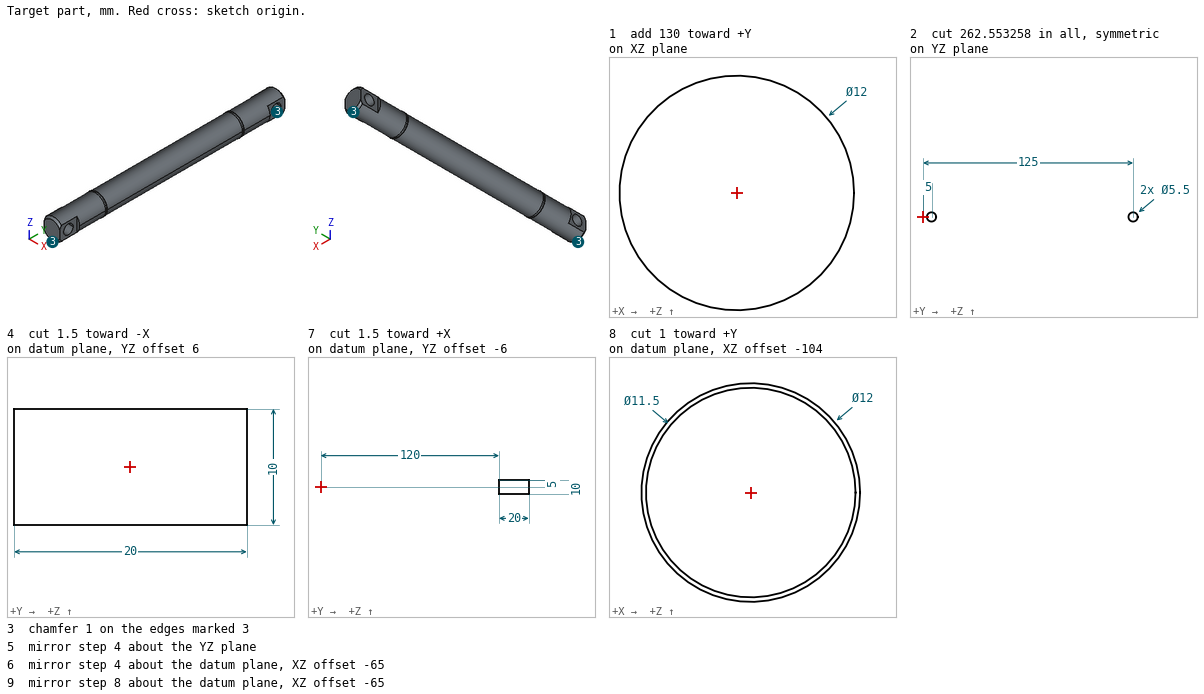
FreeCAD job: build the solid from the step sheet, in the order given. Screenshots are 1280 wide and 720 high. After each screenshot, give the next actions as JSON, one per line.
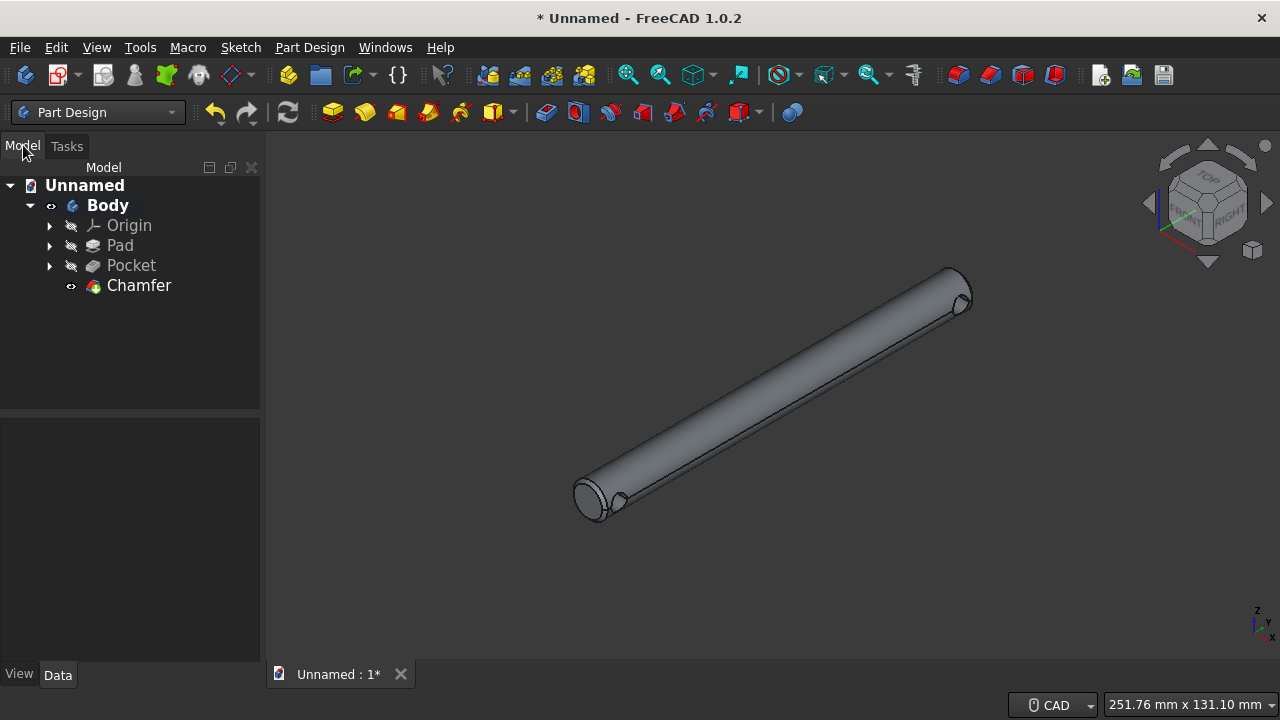
{"action": "left_click", "coordinate": [50, 226]}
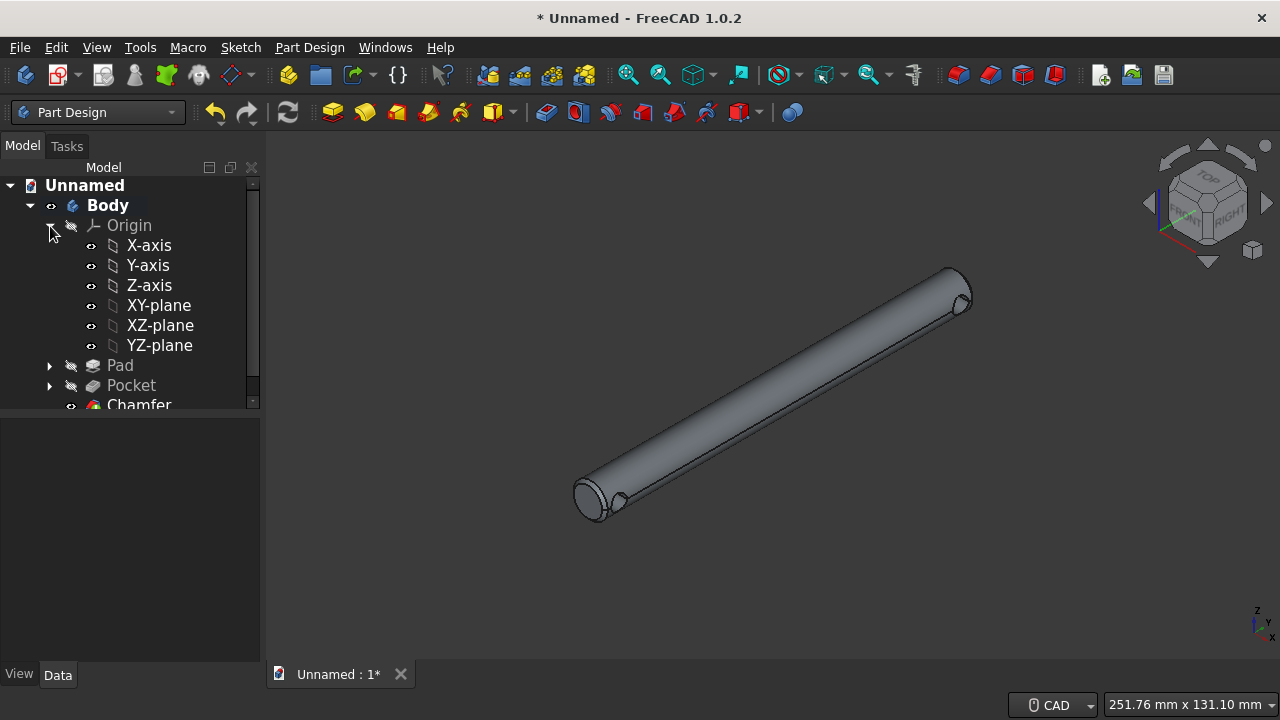
{"action": "left_click", "coordinate": [136, 346]}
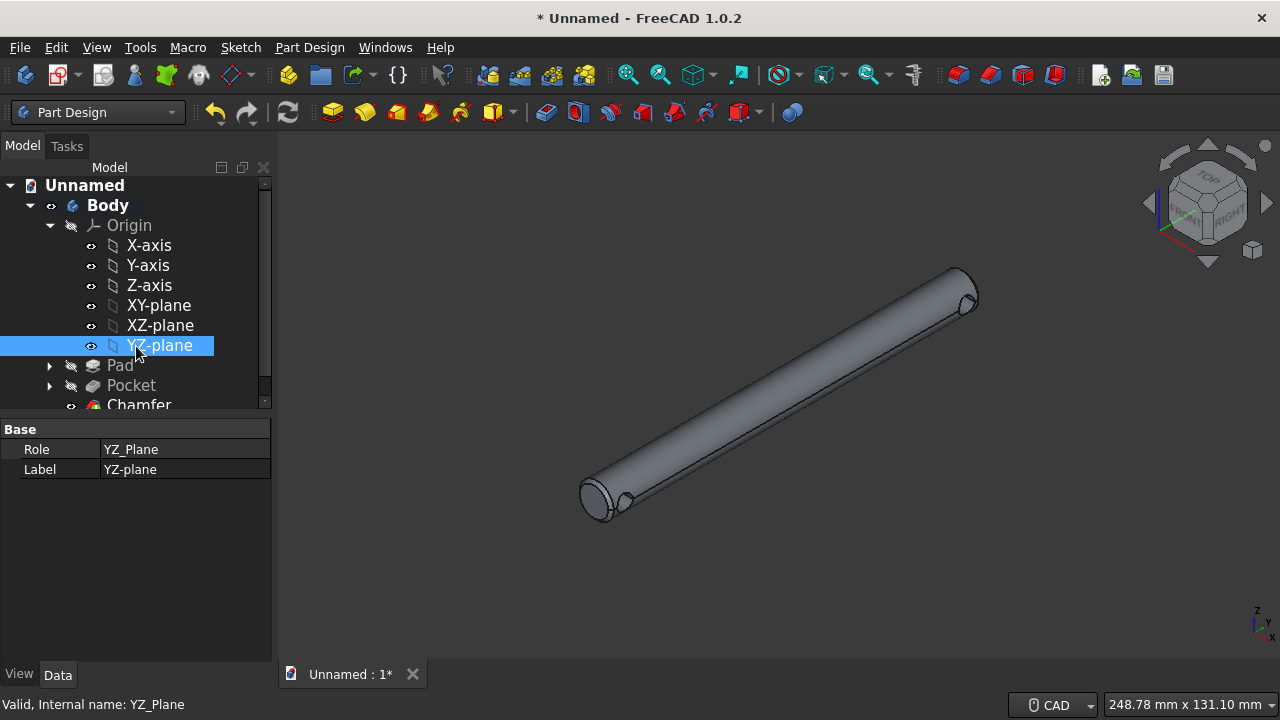
{"action": "left_click", "coordinate": [232, 76]}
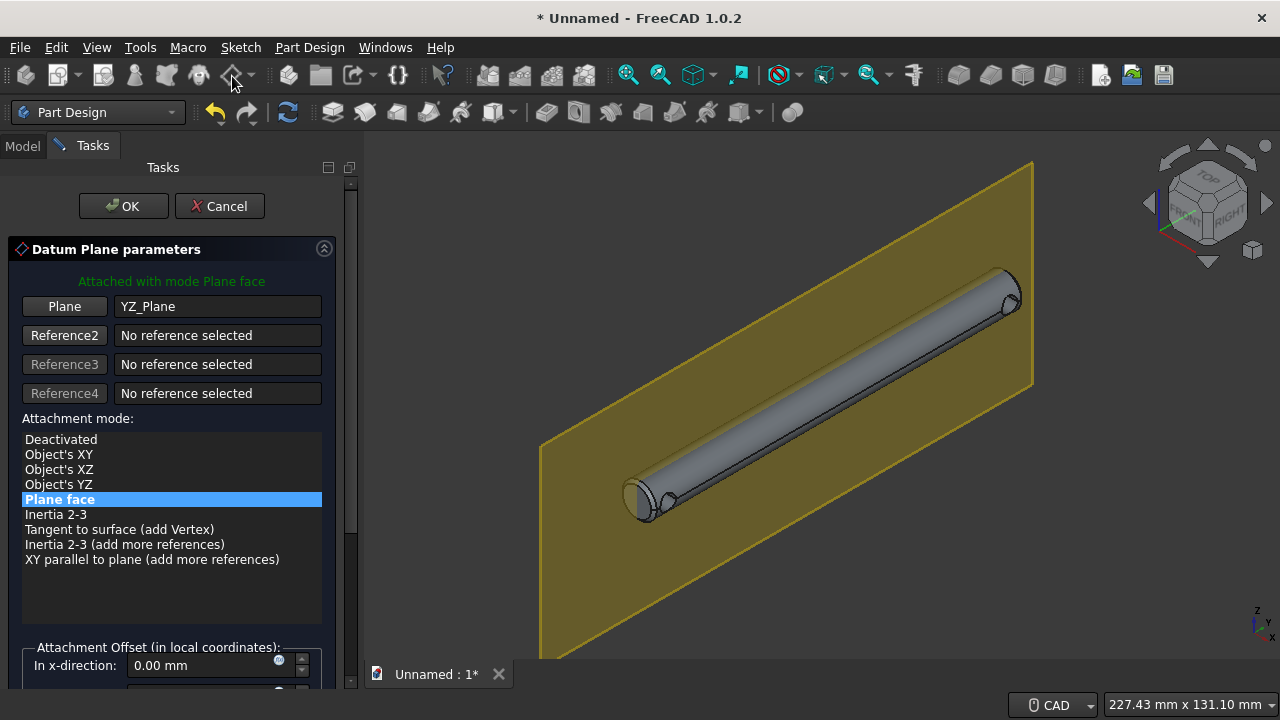
{"action": "scroll", "coordinate": [351, 432], "scroll_direction": "down", "scroll_amount": 2}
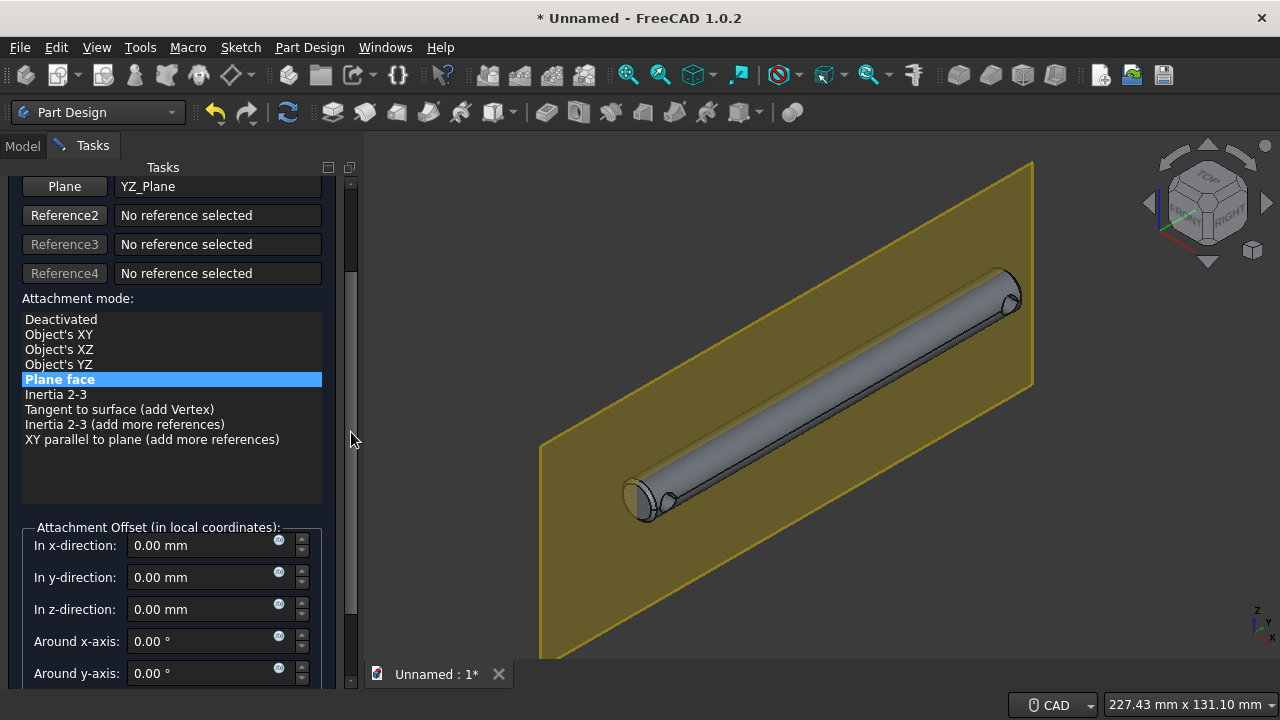
{"action": "triple_click", "coordinate": [210, 609]}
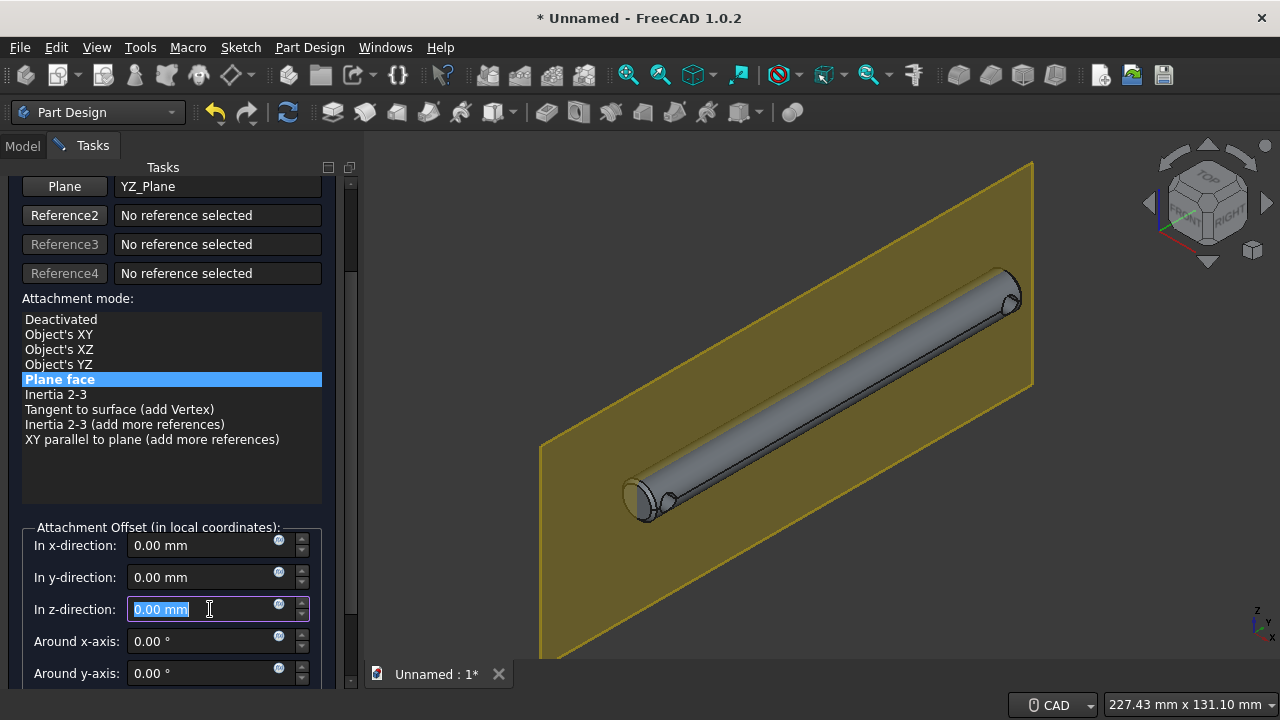
{"action": "type", "text": "6"}
{"action": "key", "text": "Tab"}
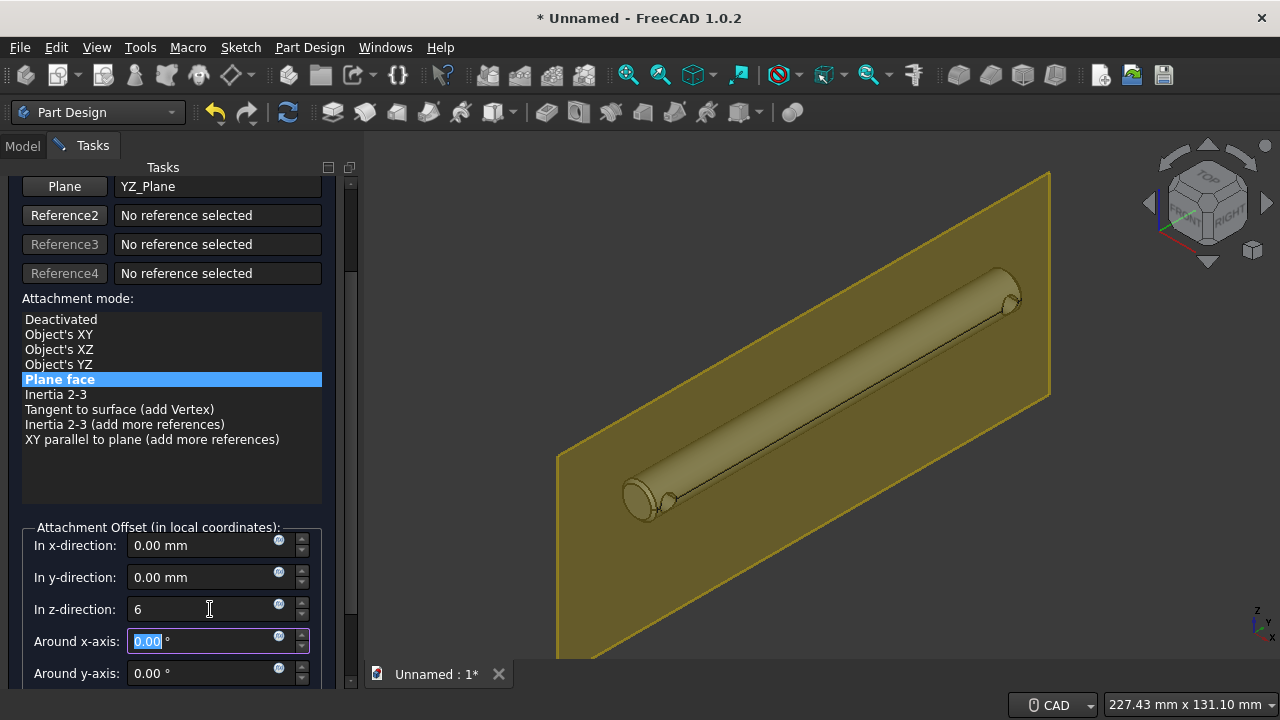
{"action": "scroll", "coordinate": [351, 432], "scroll_direction": "up", "scroll_amount": 3}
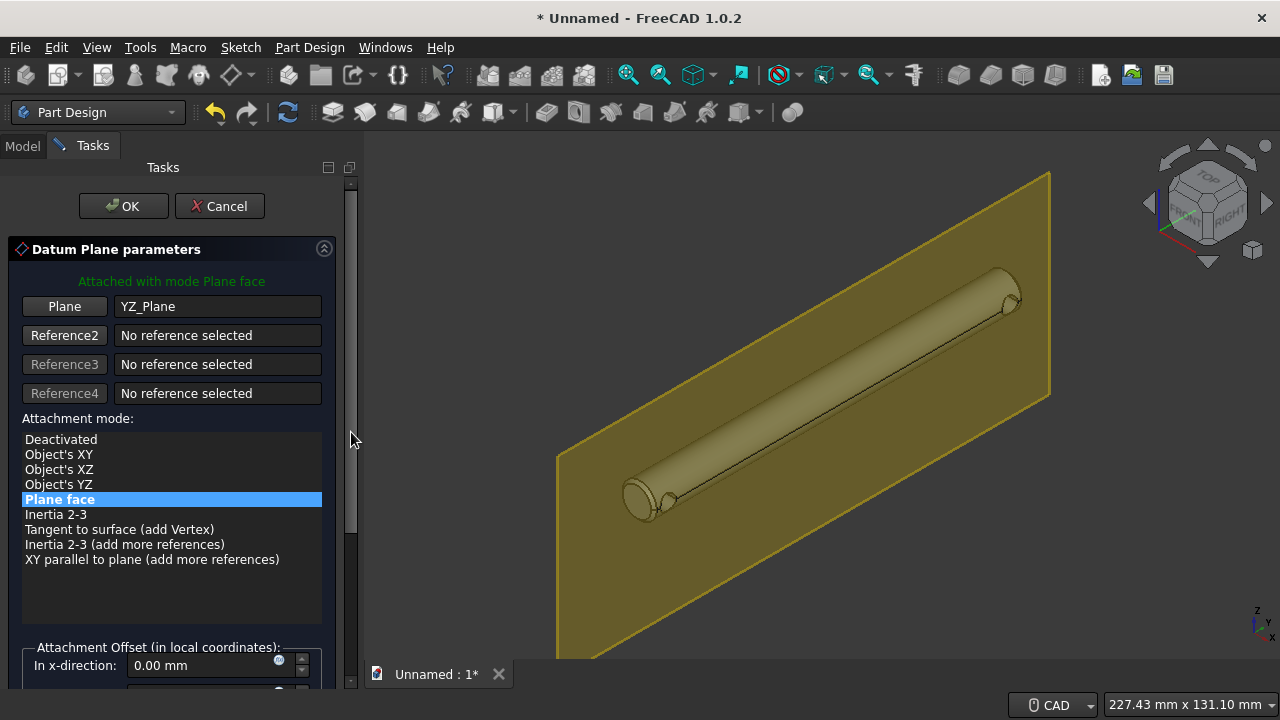
{"action": "left_click", "coordinate": [124, 206]}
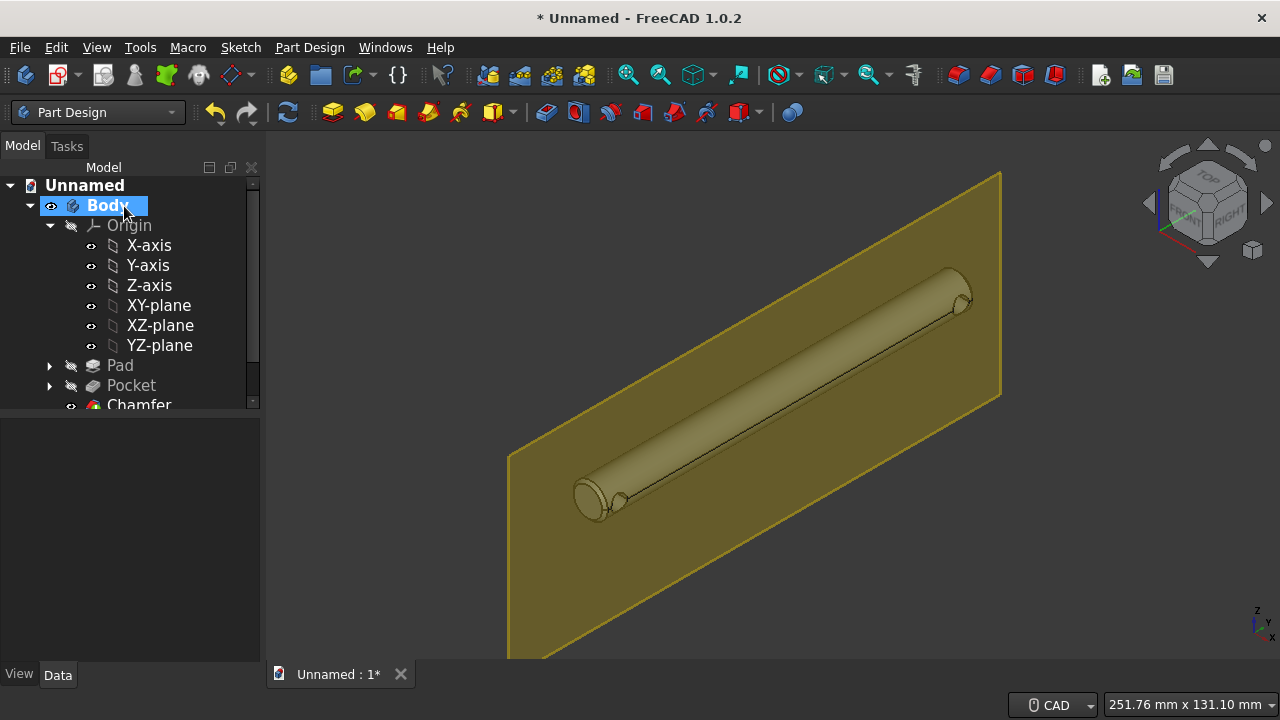
{"action": "scroll", "coordinate": [100, 301], "scroll_direction": "down", "scroll_amount": 3}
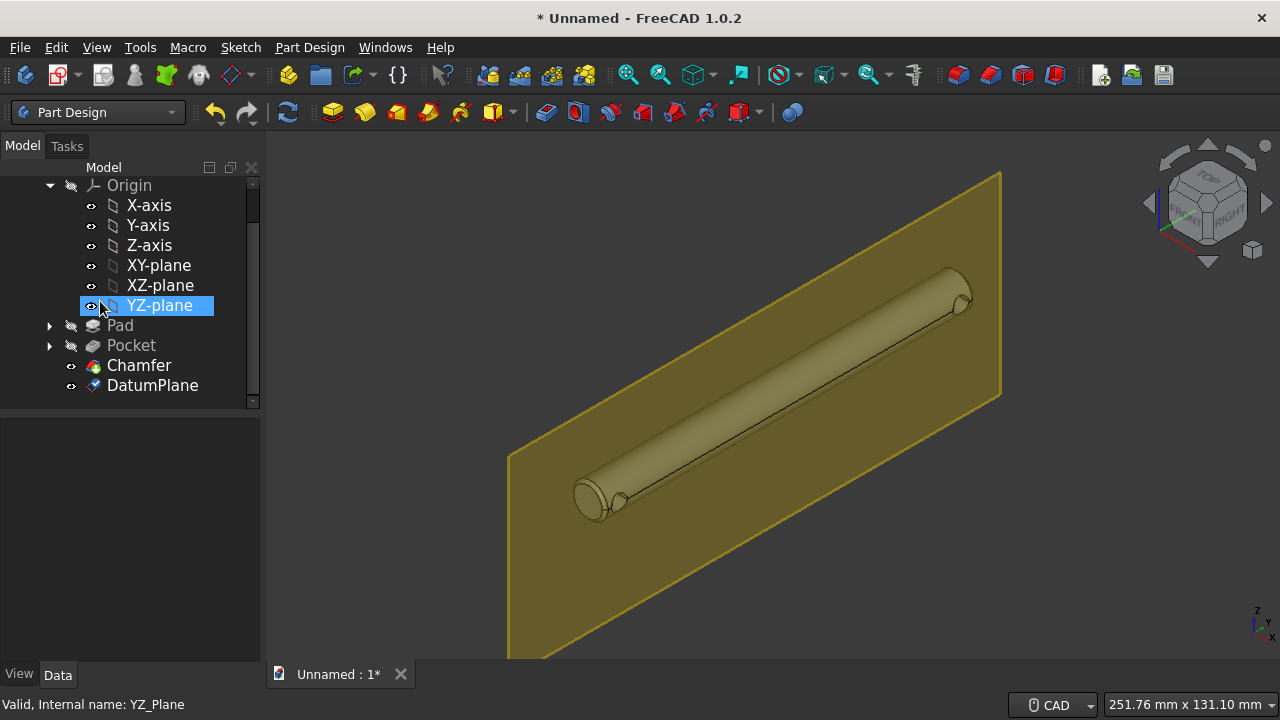
{"action": "left_click", "coordinate": [116, 386]}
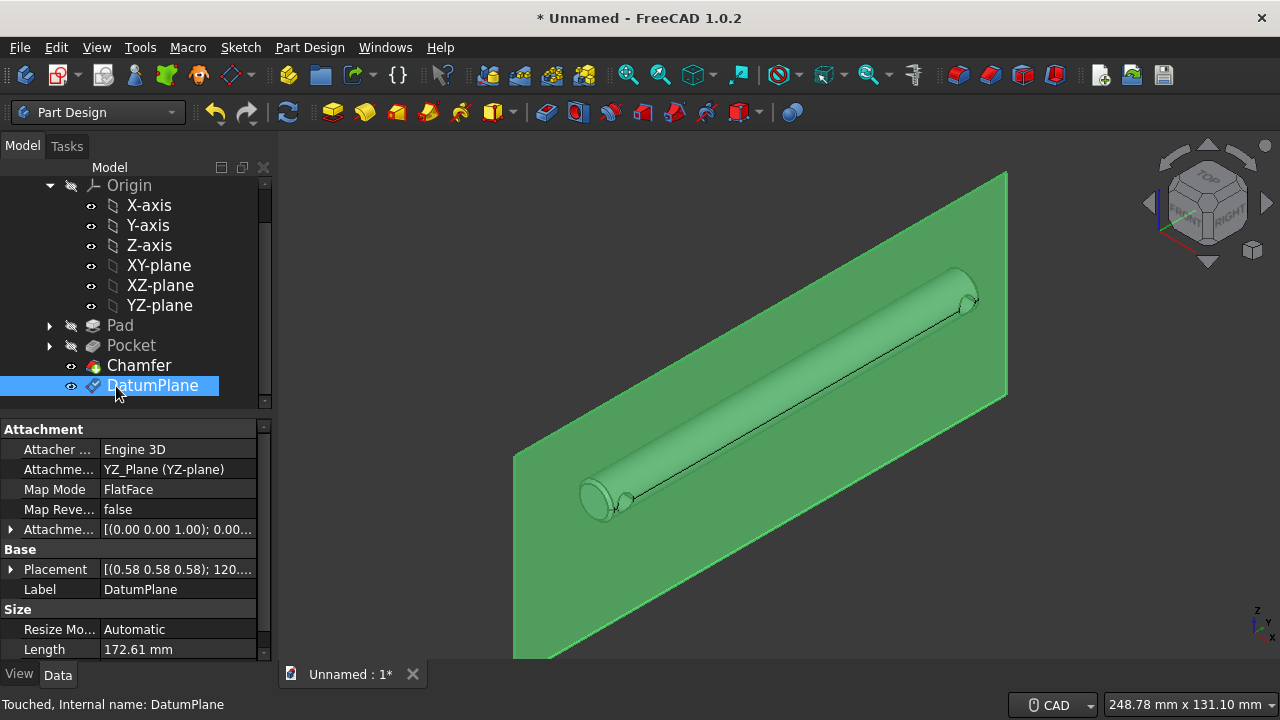
{"action": "left_click", "coordinate": [58, 76]}